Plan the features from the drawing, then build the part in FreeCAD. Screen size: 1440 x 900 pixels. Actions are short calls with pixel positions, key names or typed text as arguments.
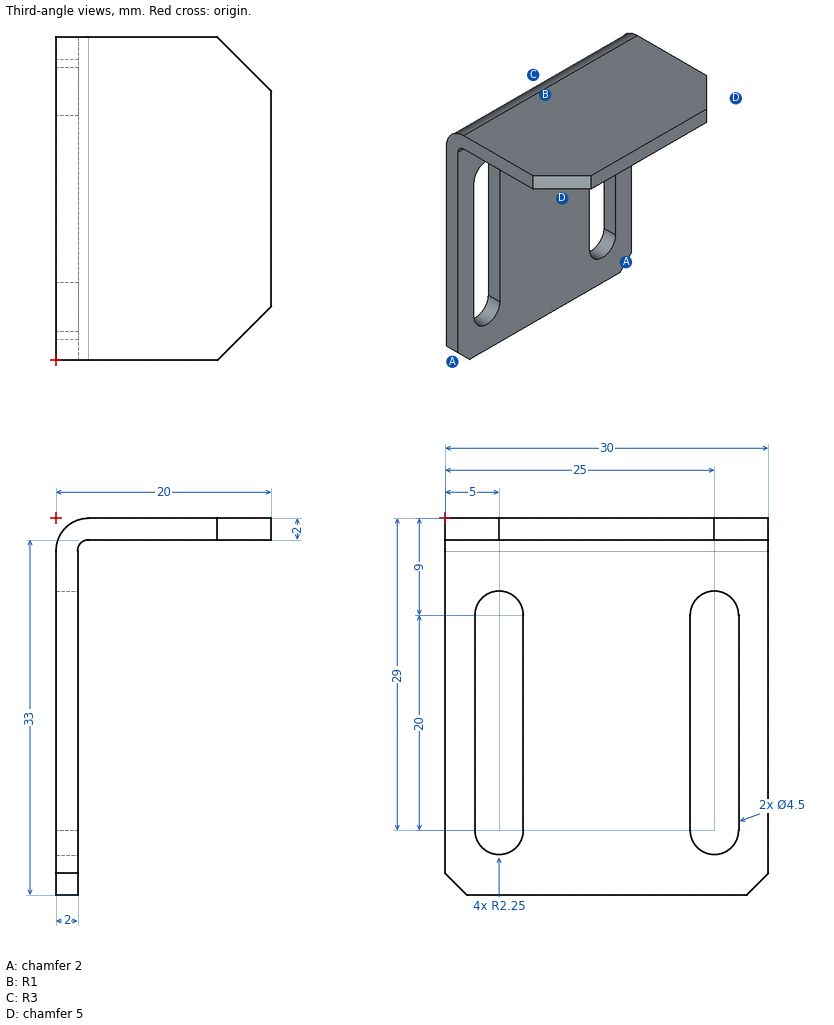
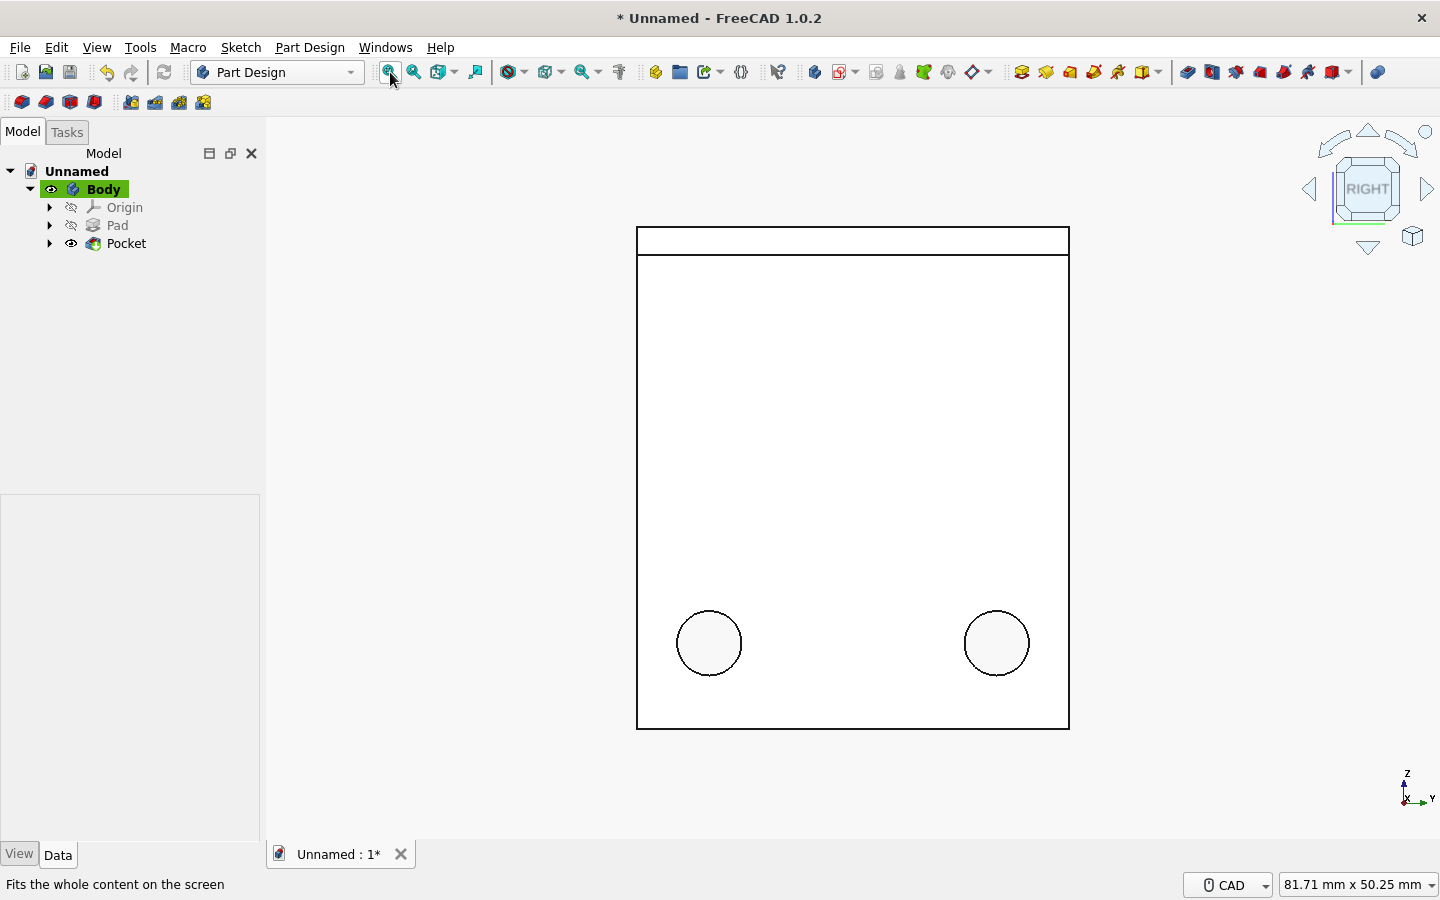
key(5)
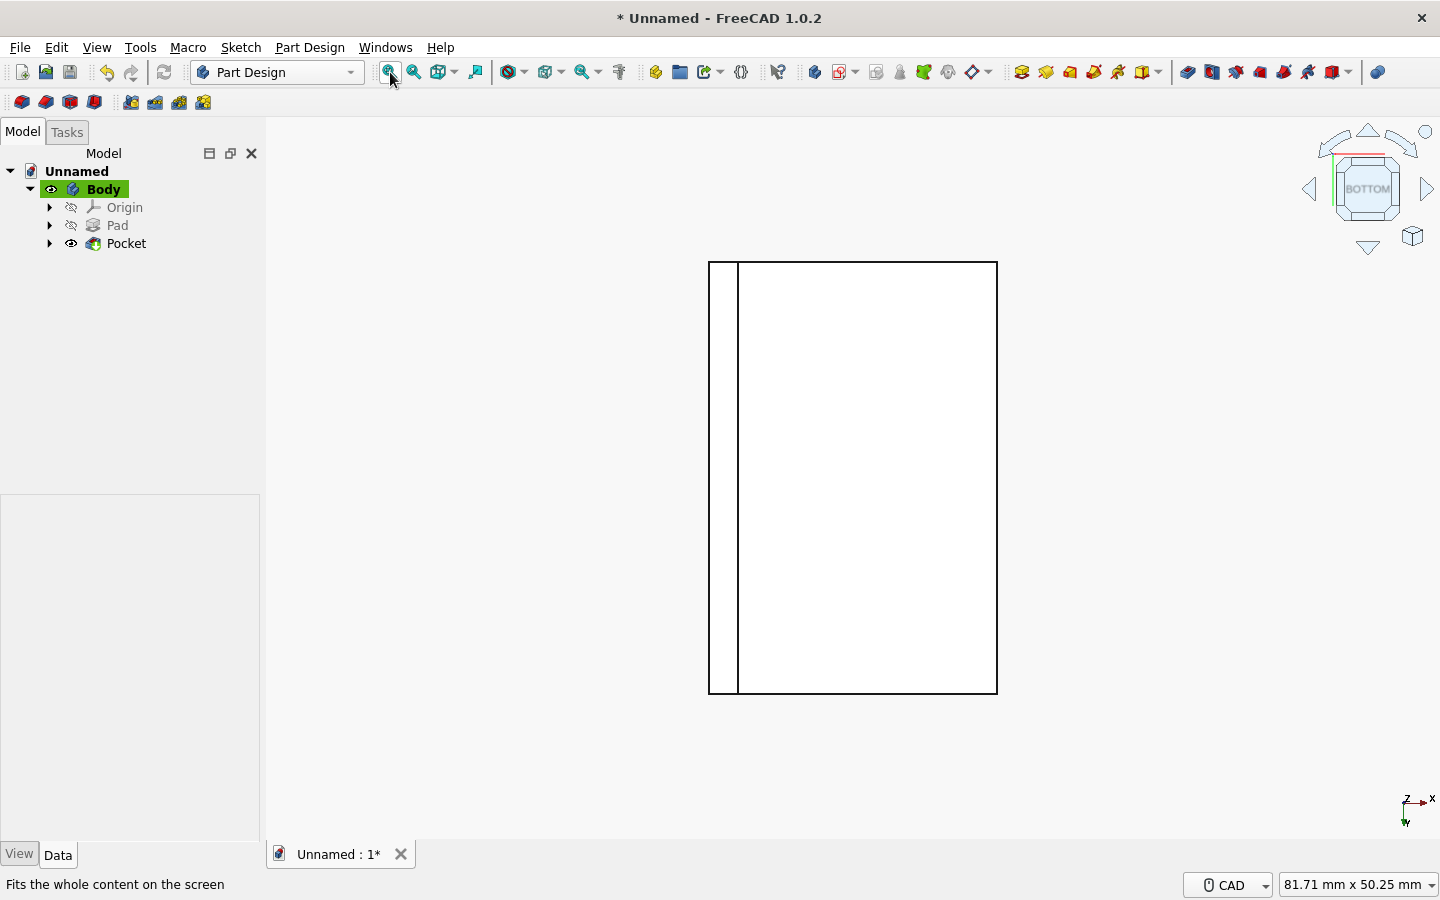
click(724, 261)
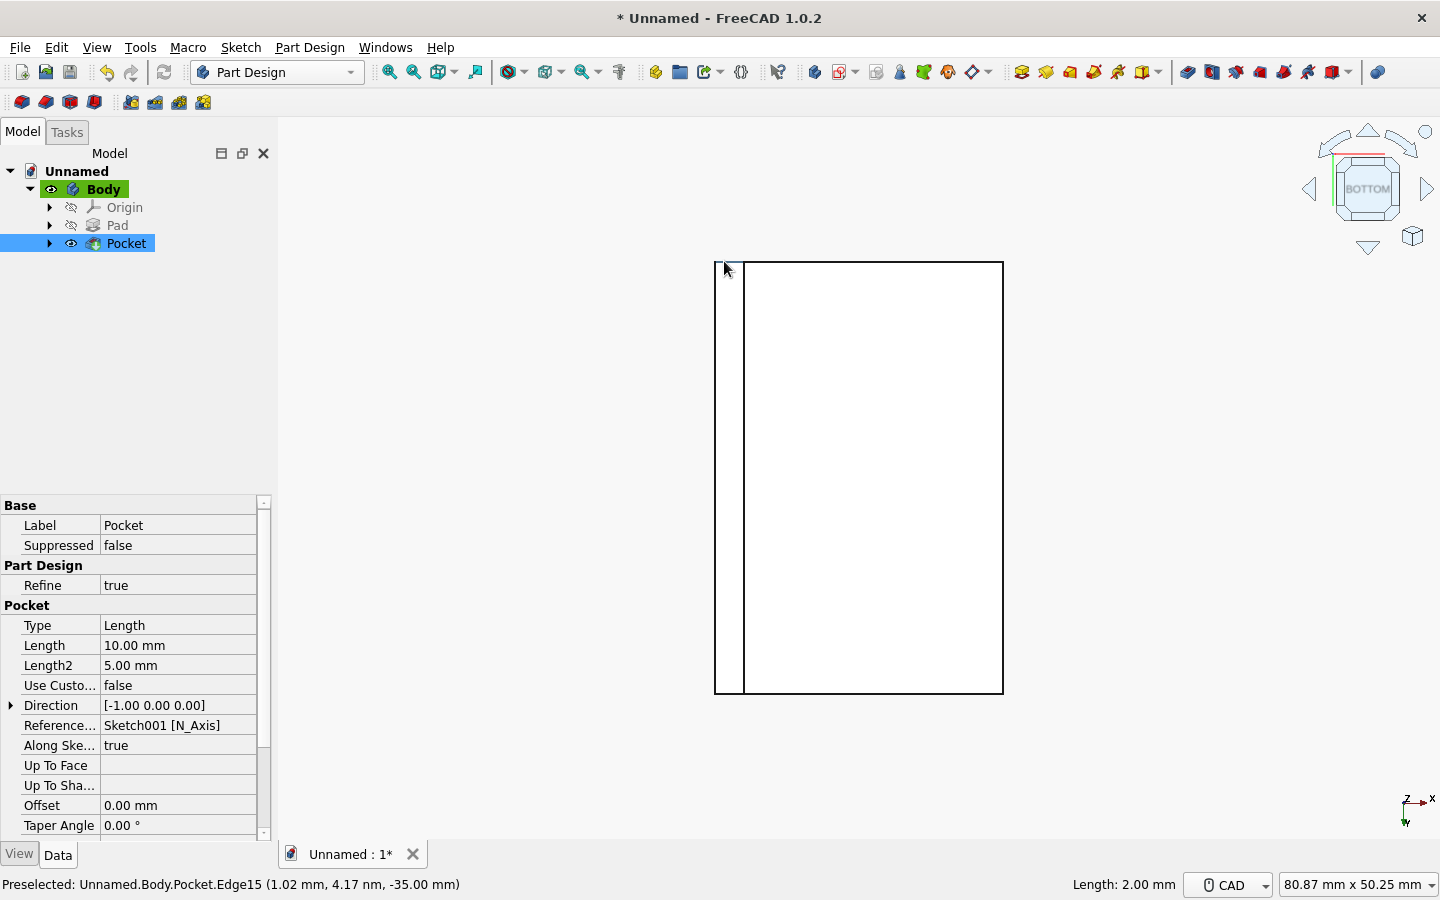
key(4)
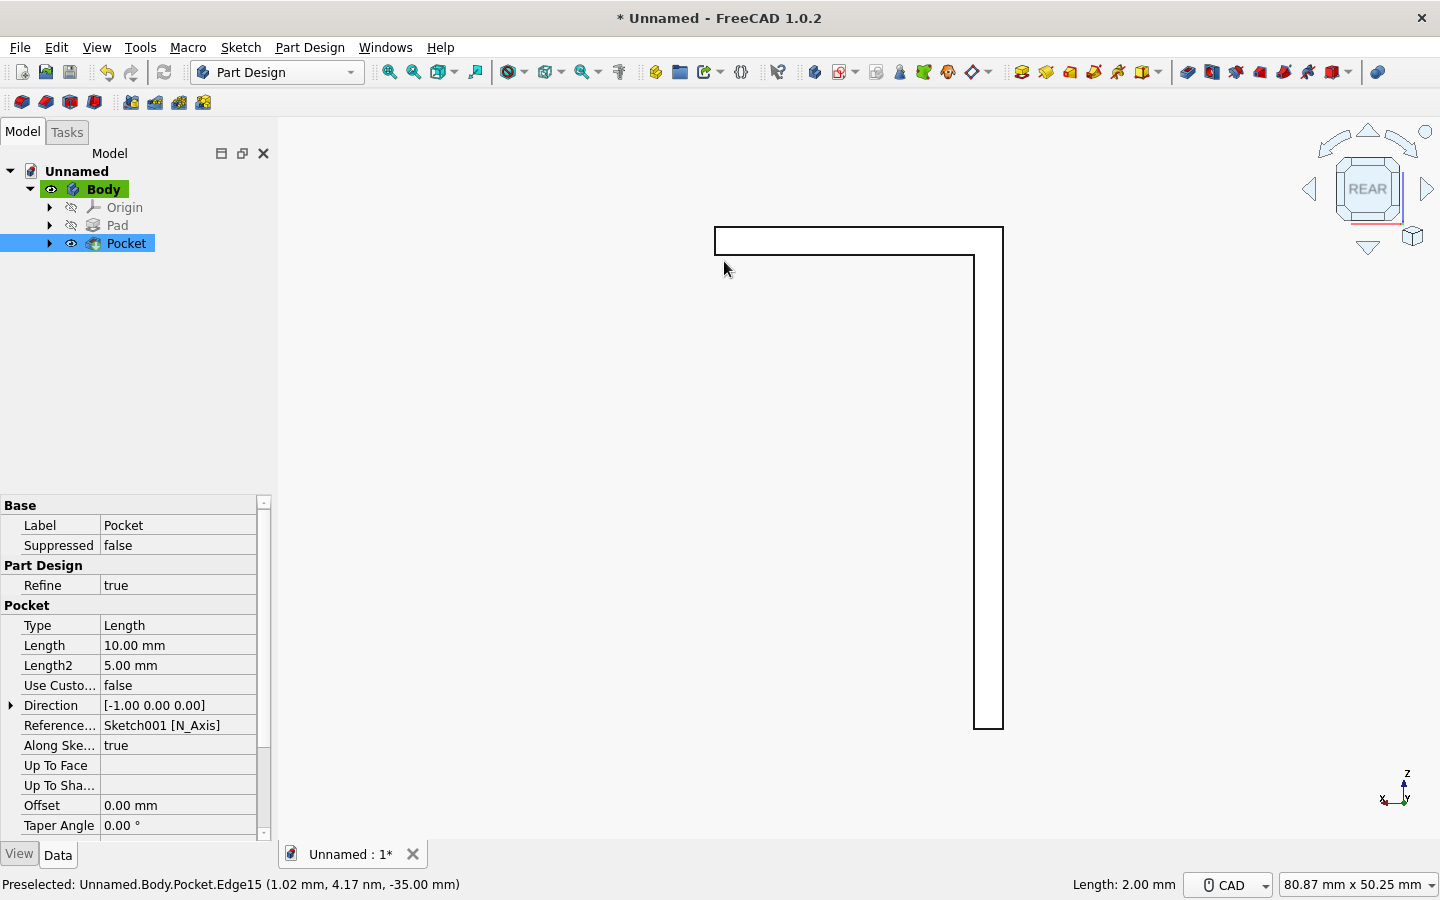
click(988, 728, ctrl)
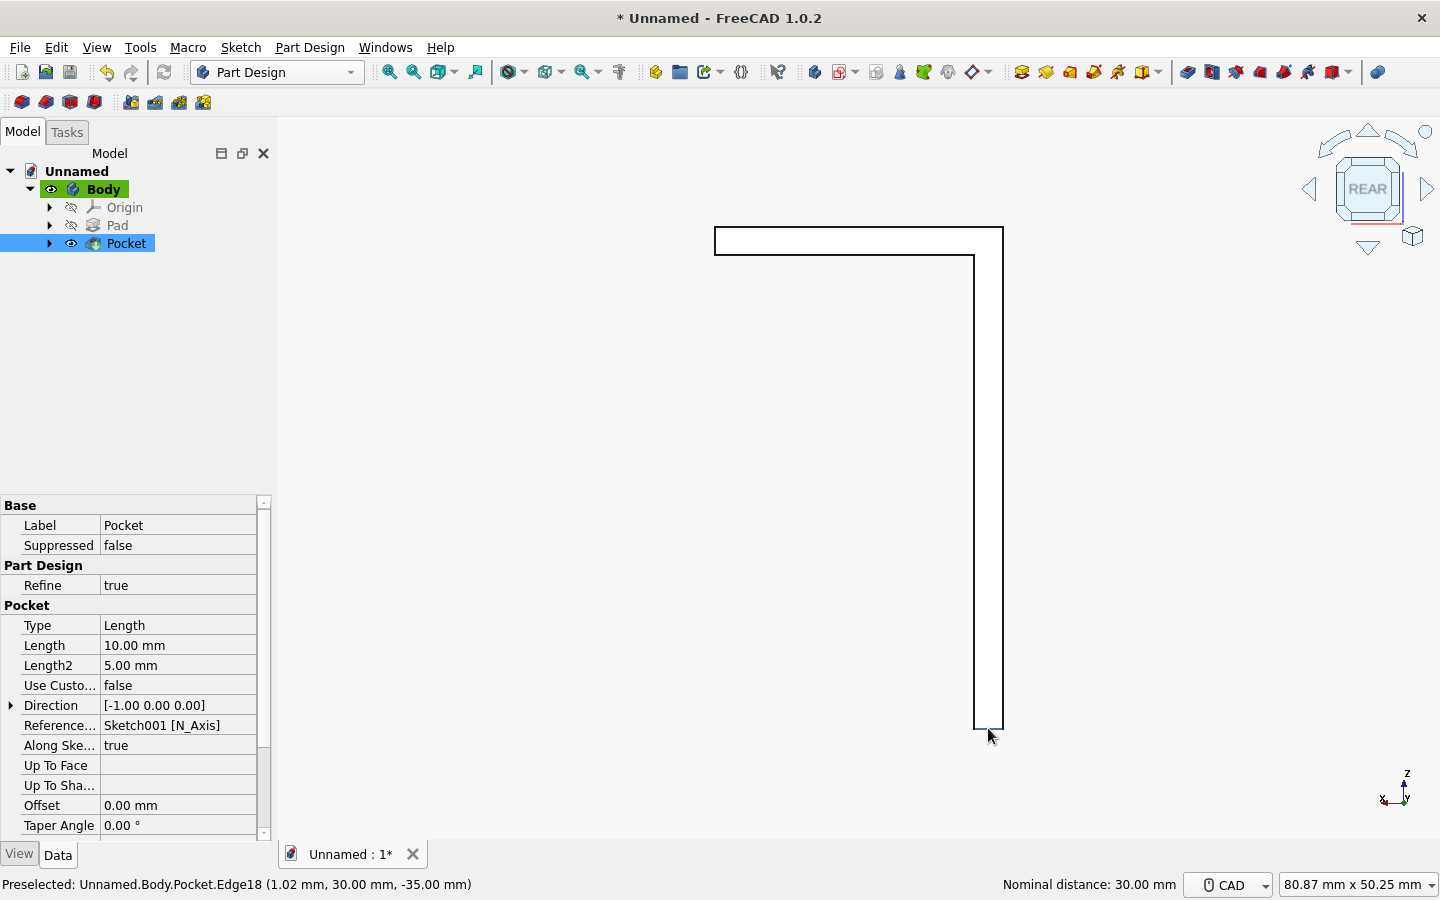
click(46, 102)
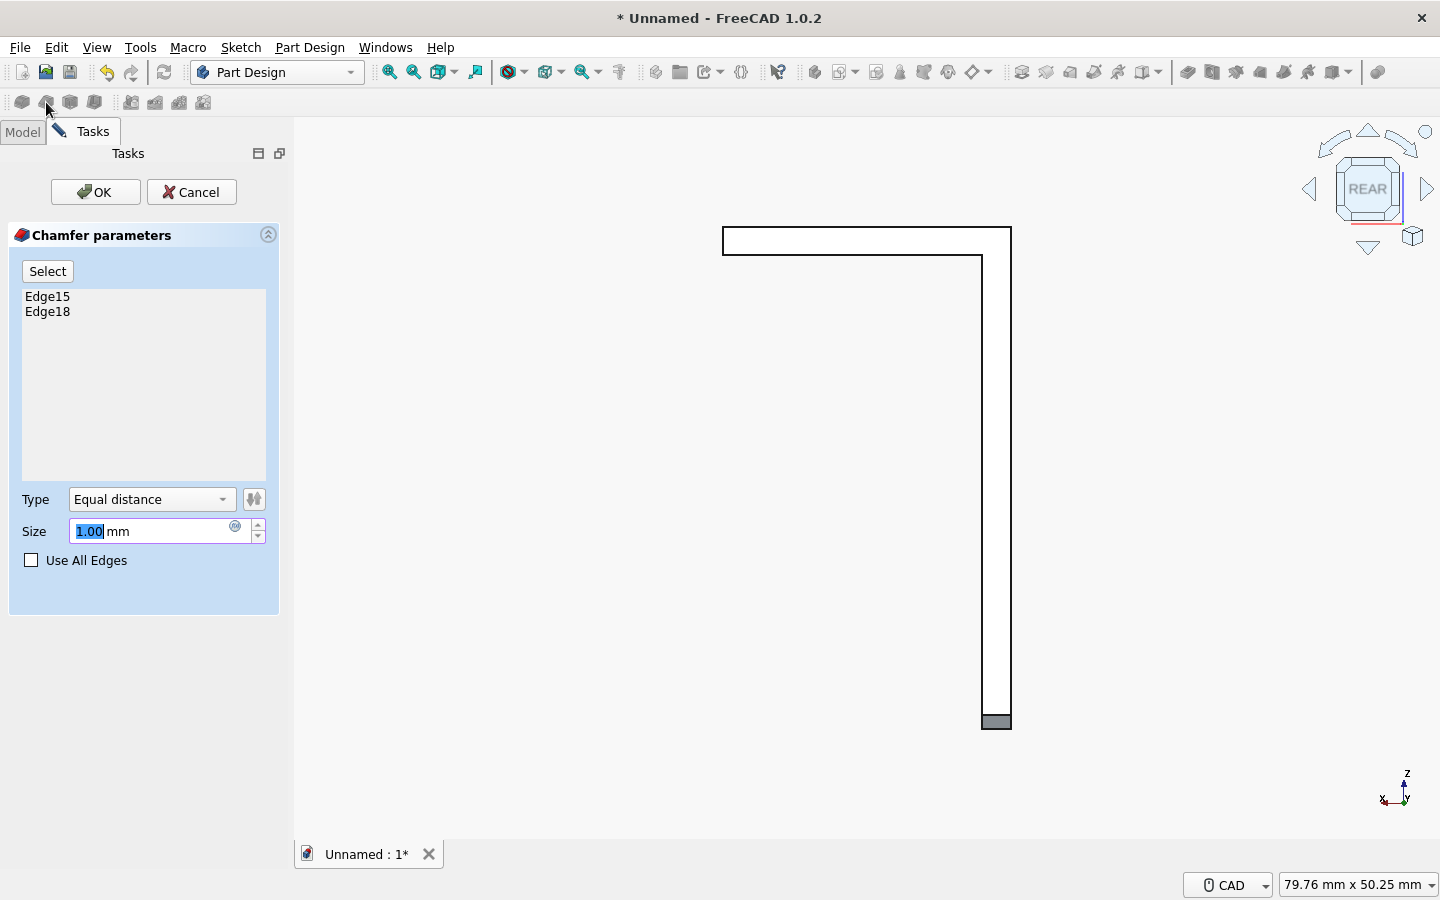
text(2)
key(Tab)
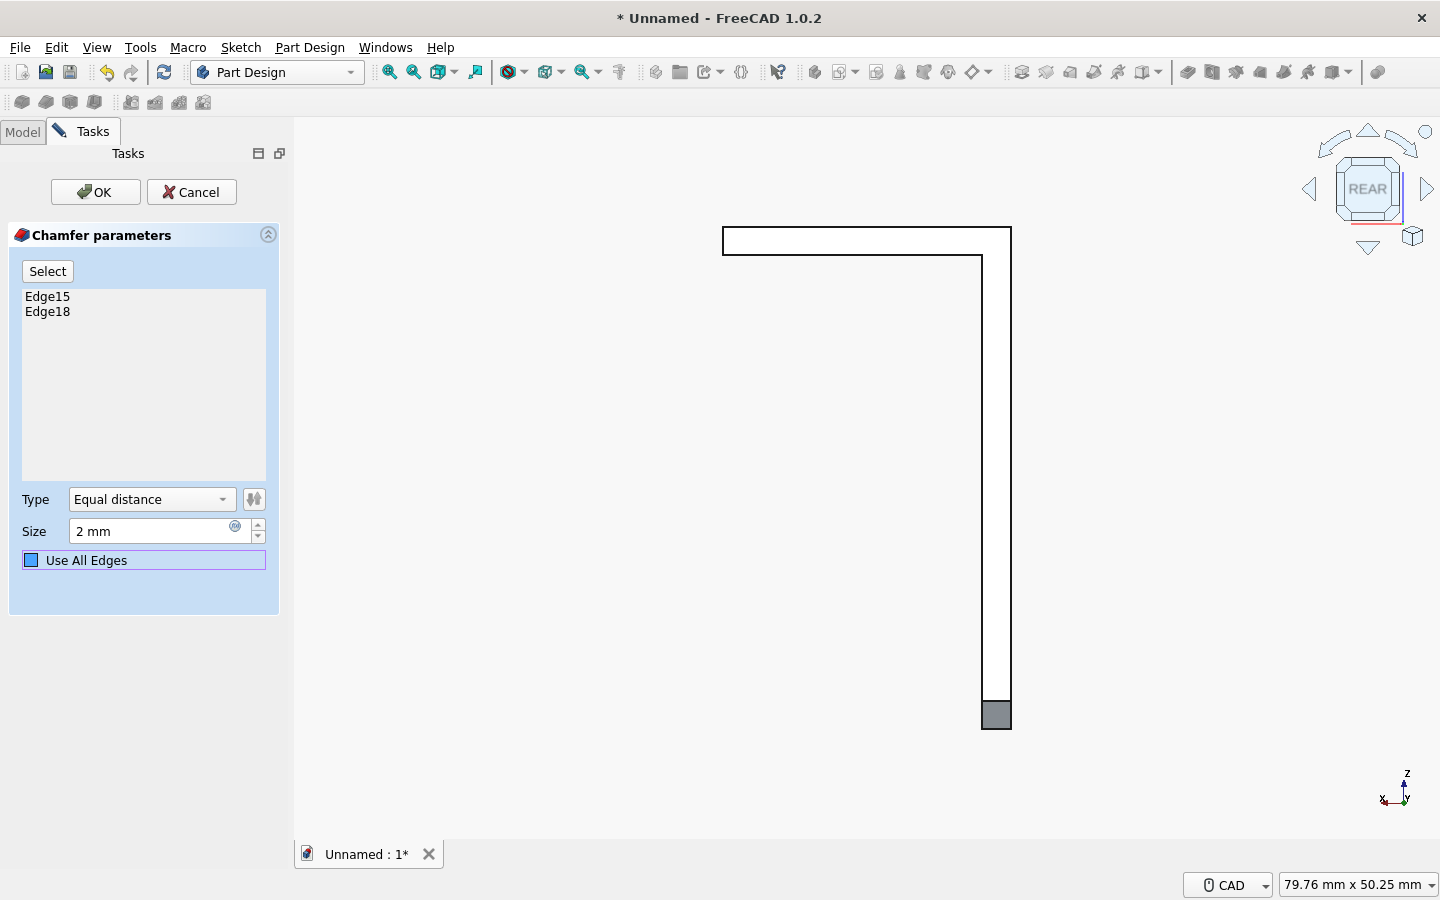
click(96, 192)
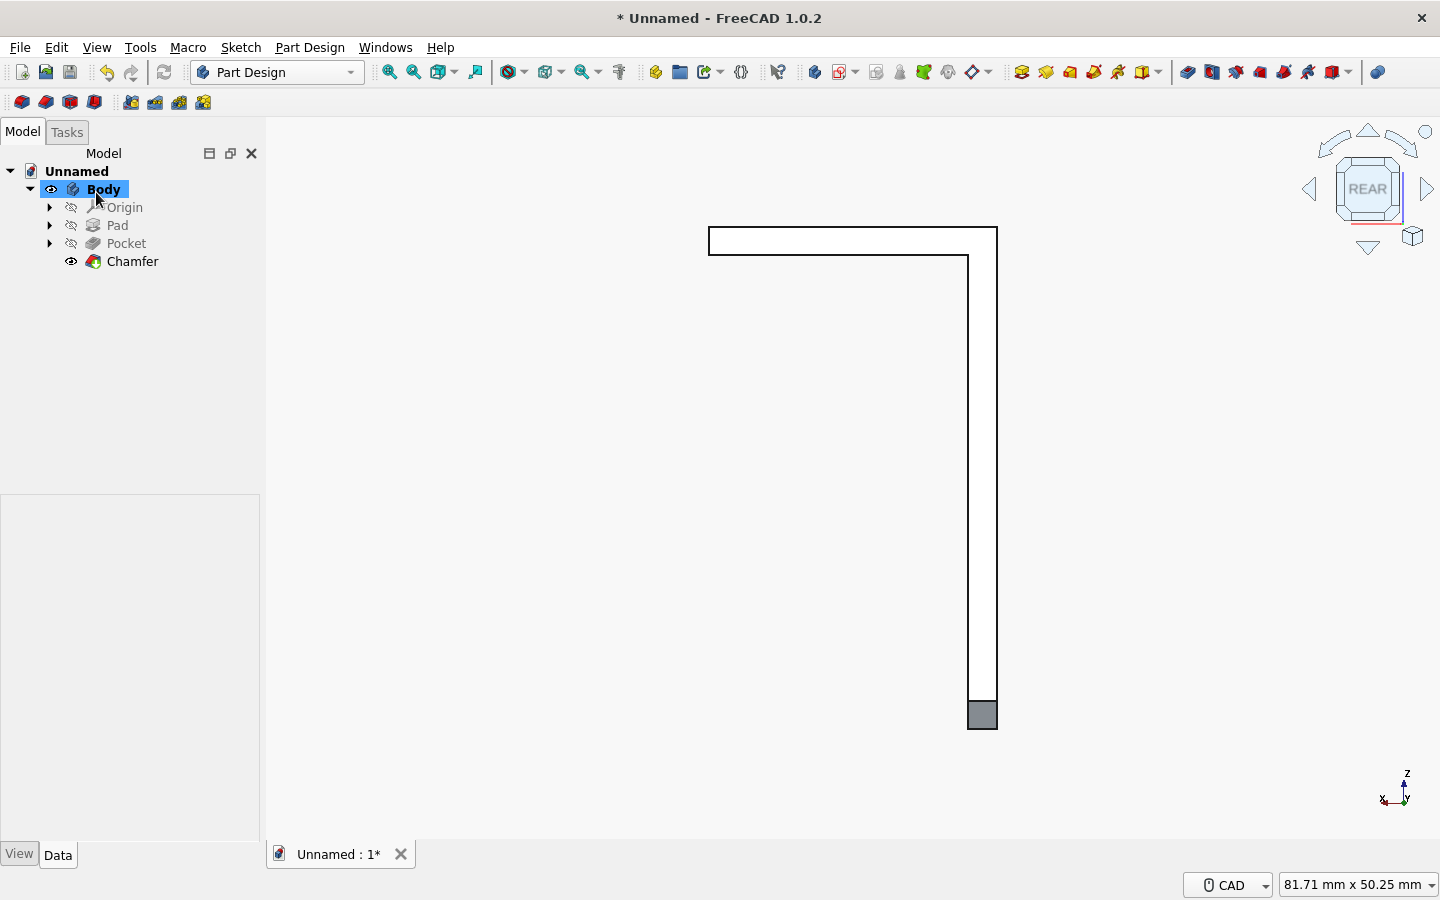
key(0)